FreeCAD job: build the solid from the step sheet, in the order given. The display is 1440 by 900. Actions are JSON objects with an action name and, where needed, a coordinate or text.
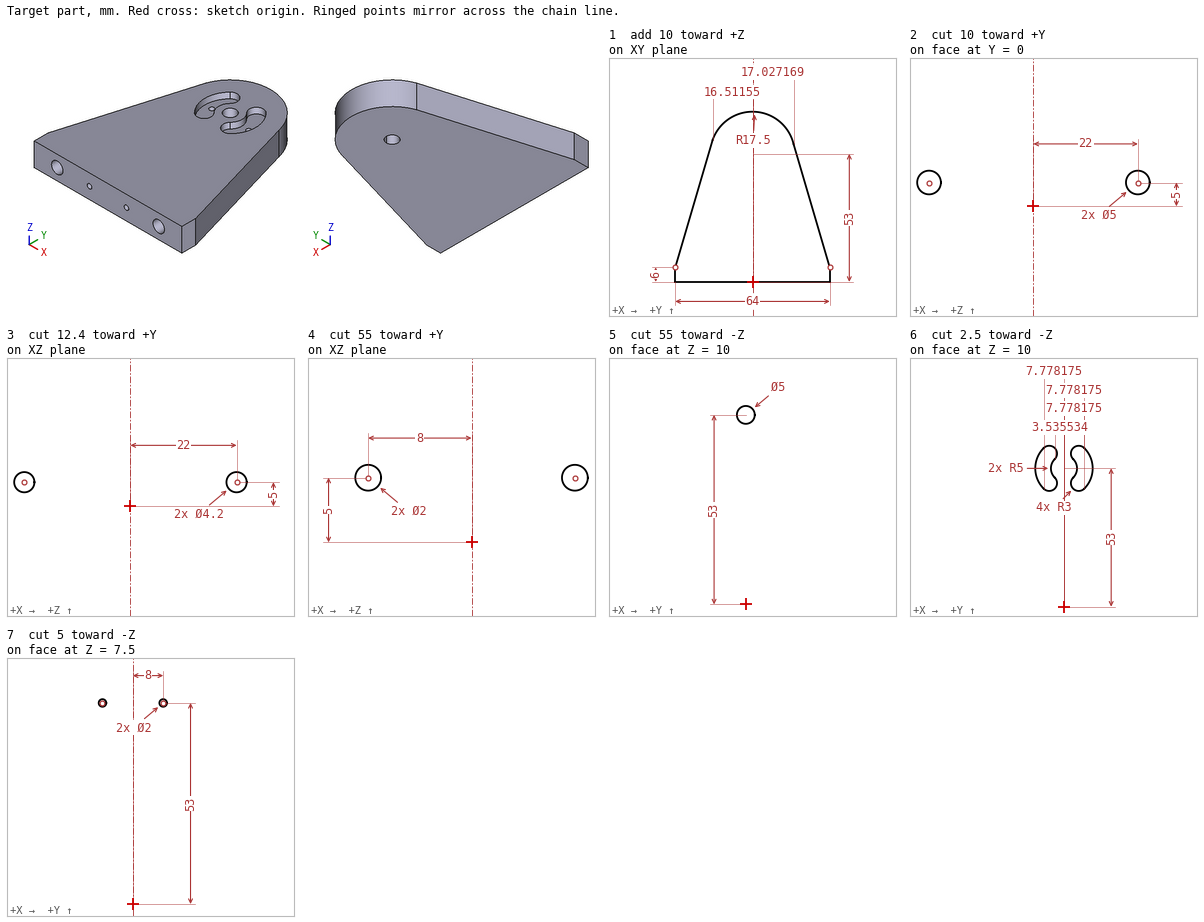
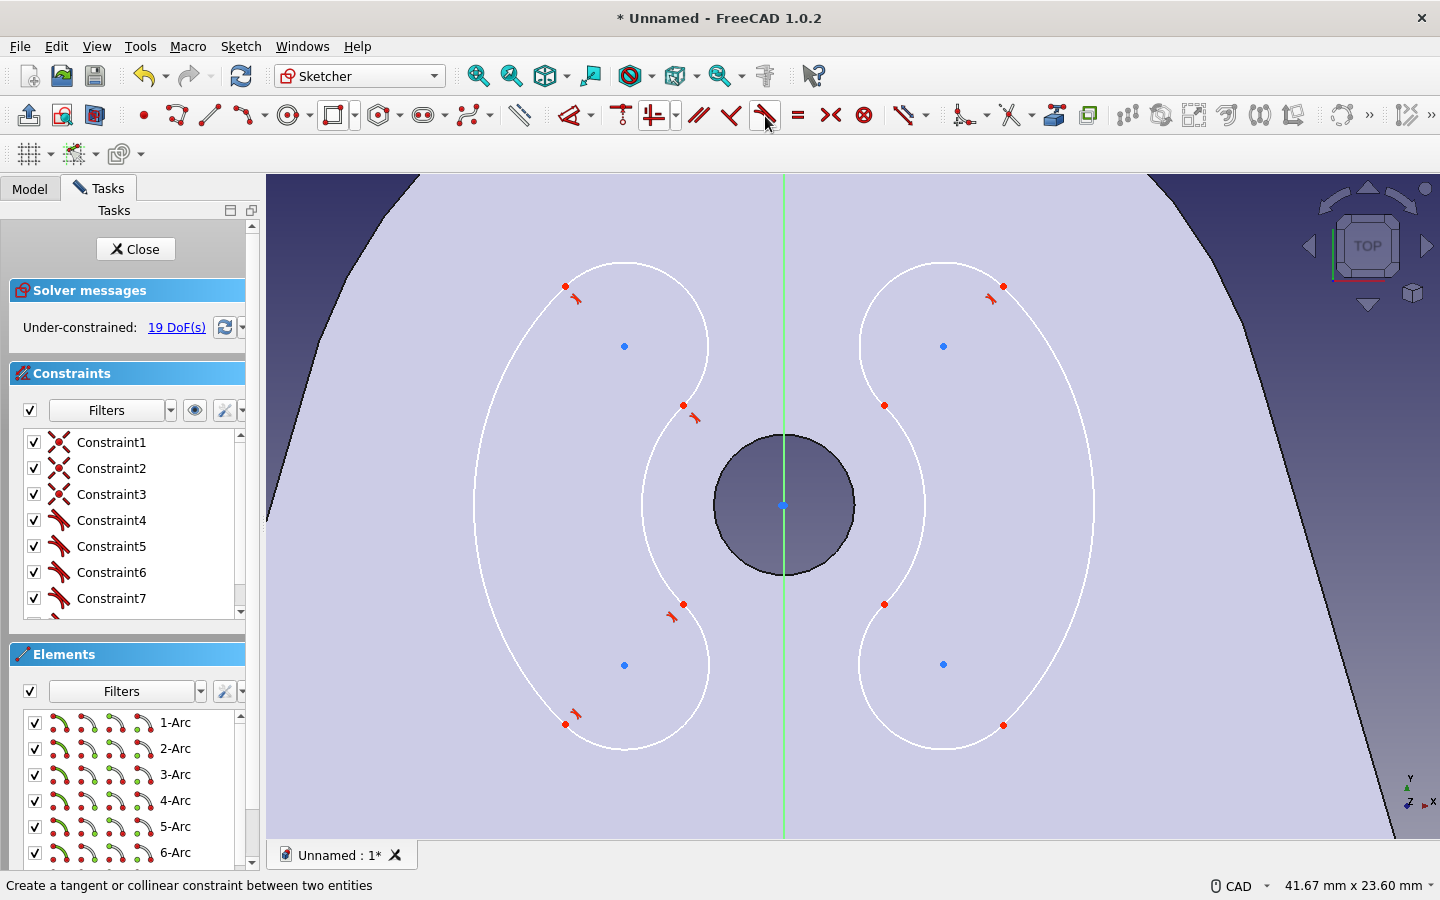
{"action": "left_click", "coordinate": [1079, 602]}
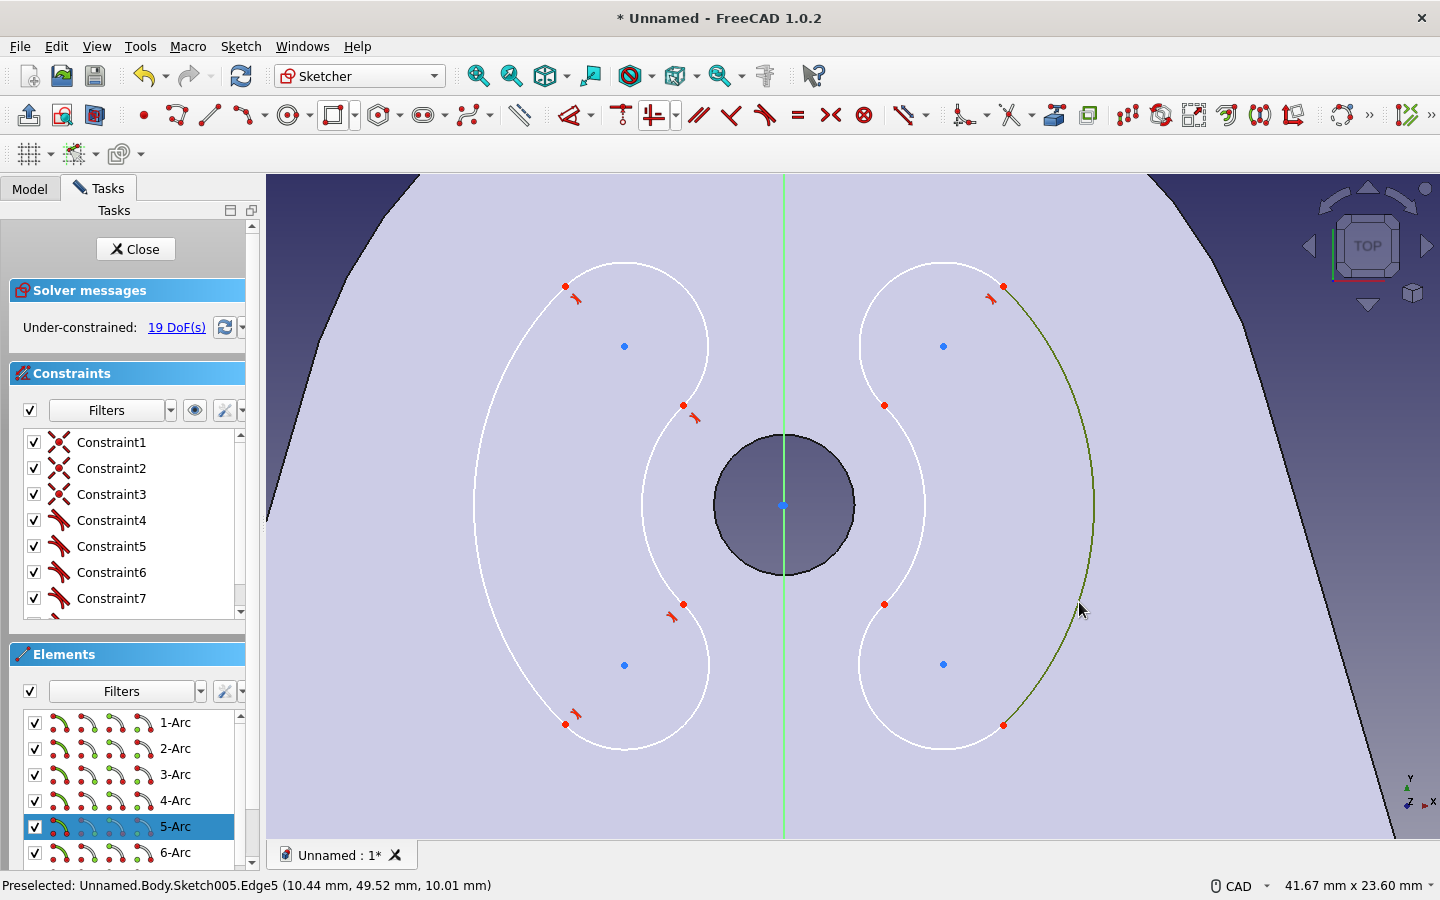
{"action": "left_click", "coordinate": [860, 678]}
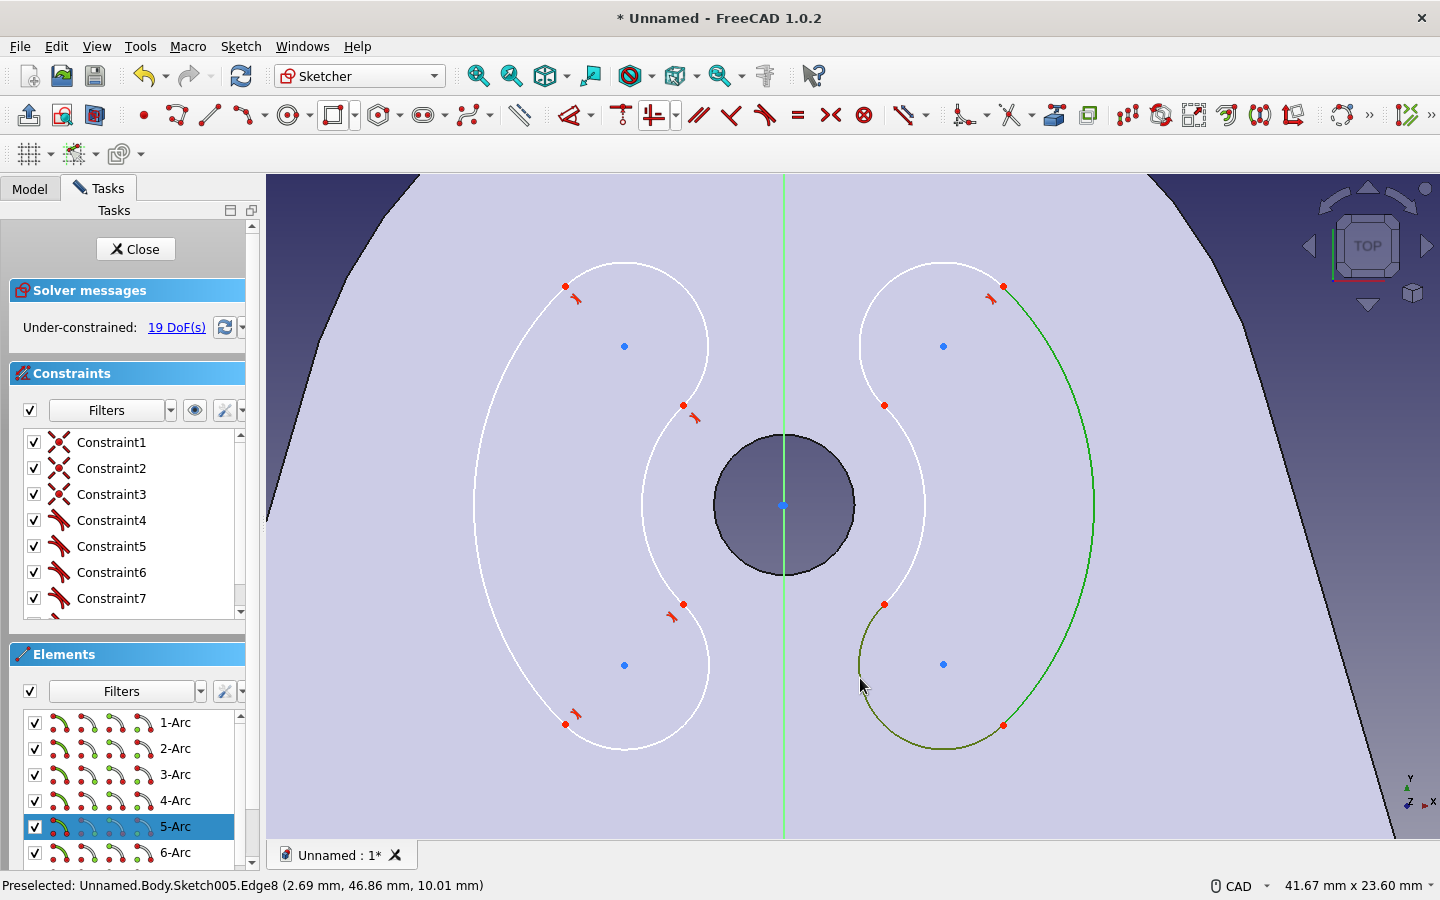
{"action": "left_click", "coordinate": [765, 116]}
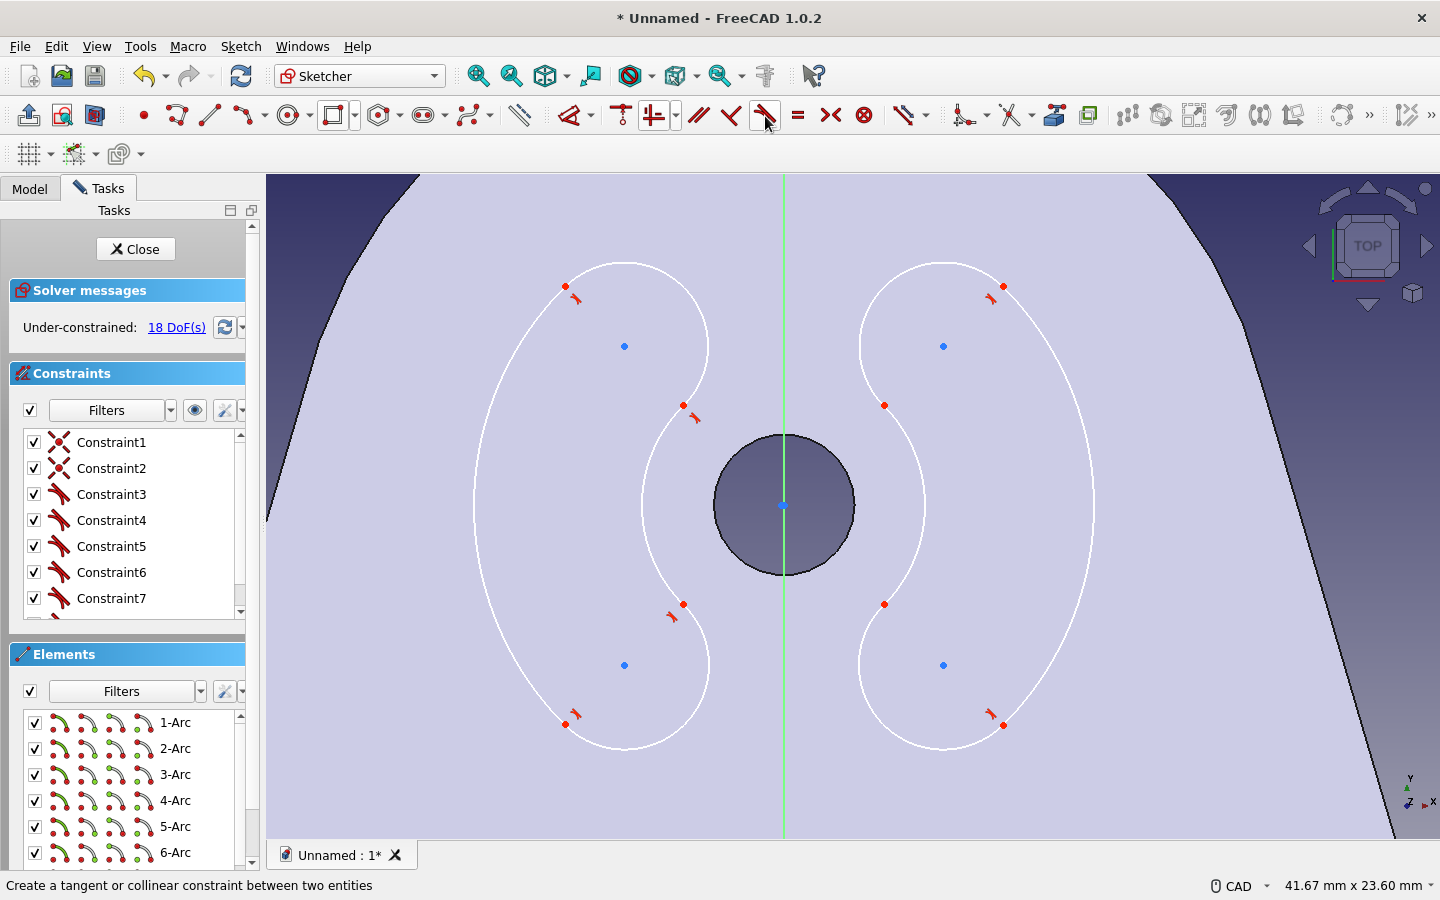
{"action": "left_click", "coordinate": [930, 264]}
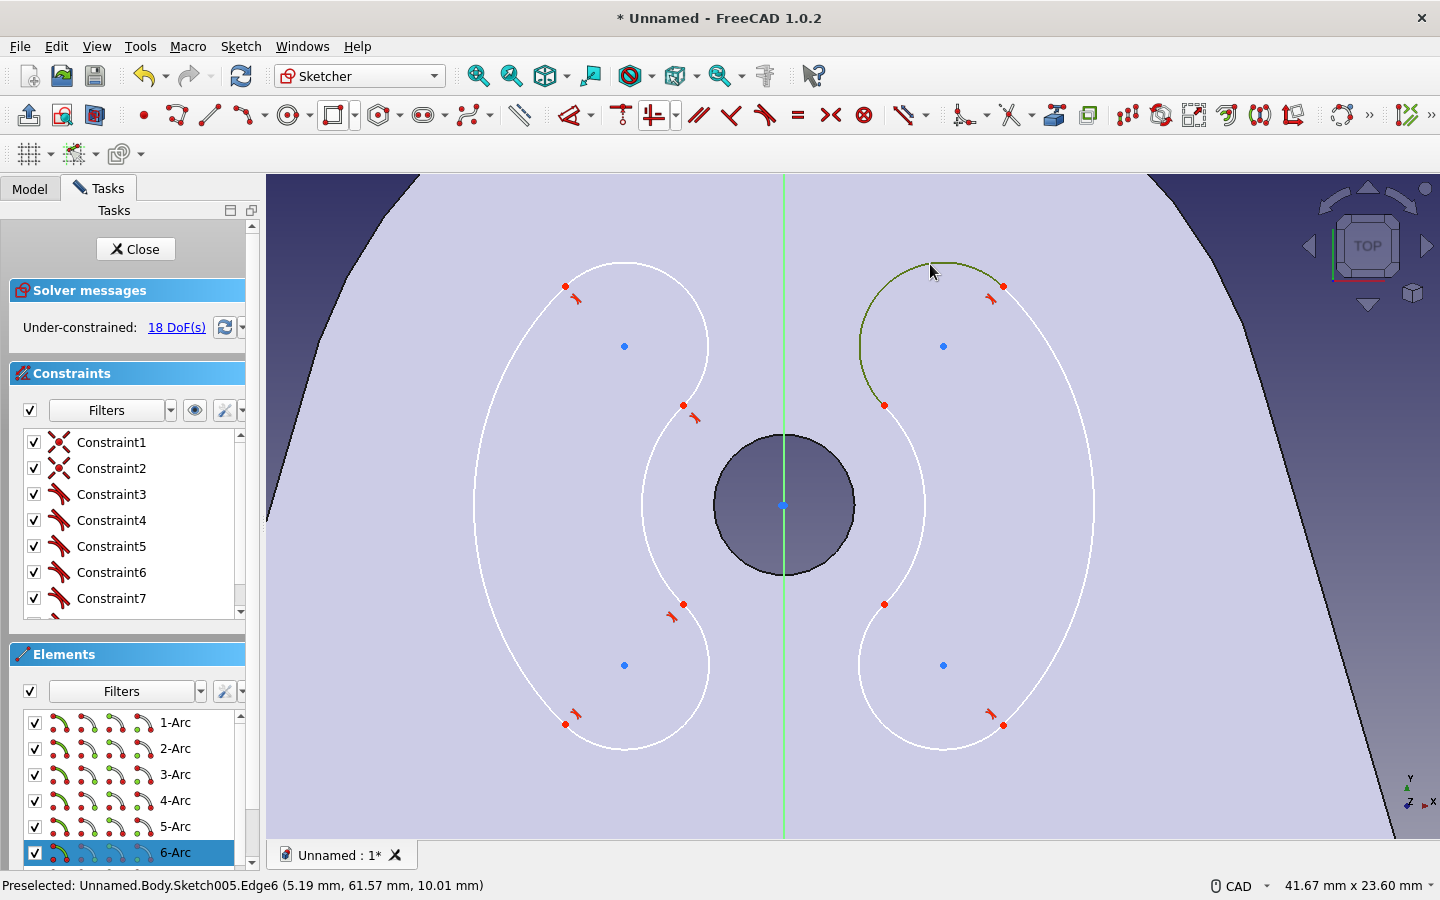
{"action": "left_click", "coordinate": [918, 549]}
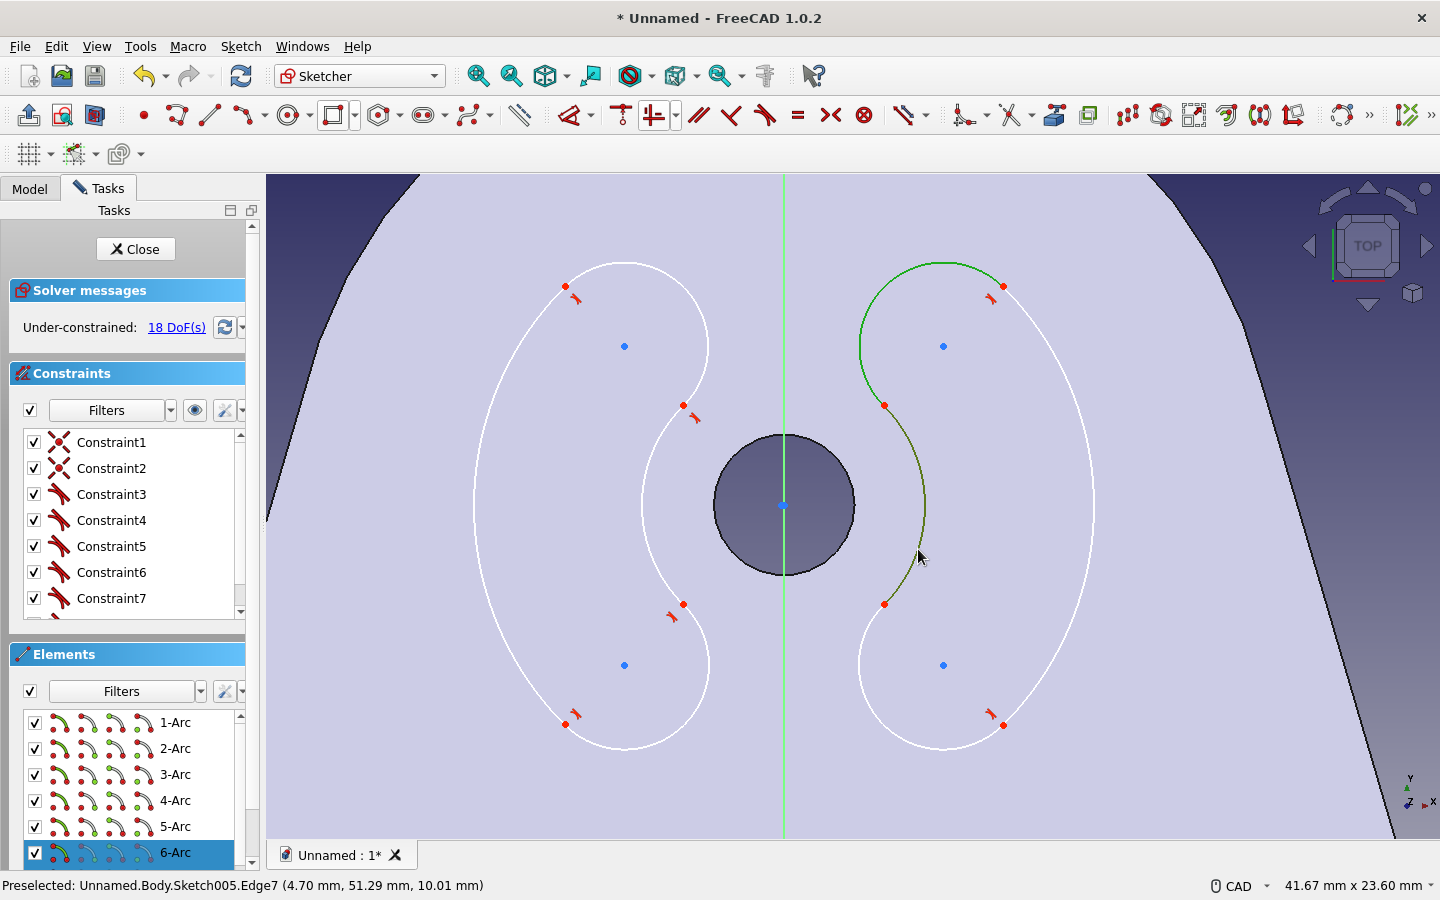
{"action": "left_click", "coordinate": [765, 116]}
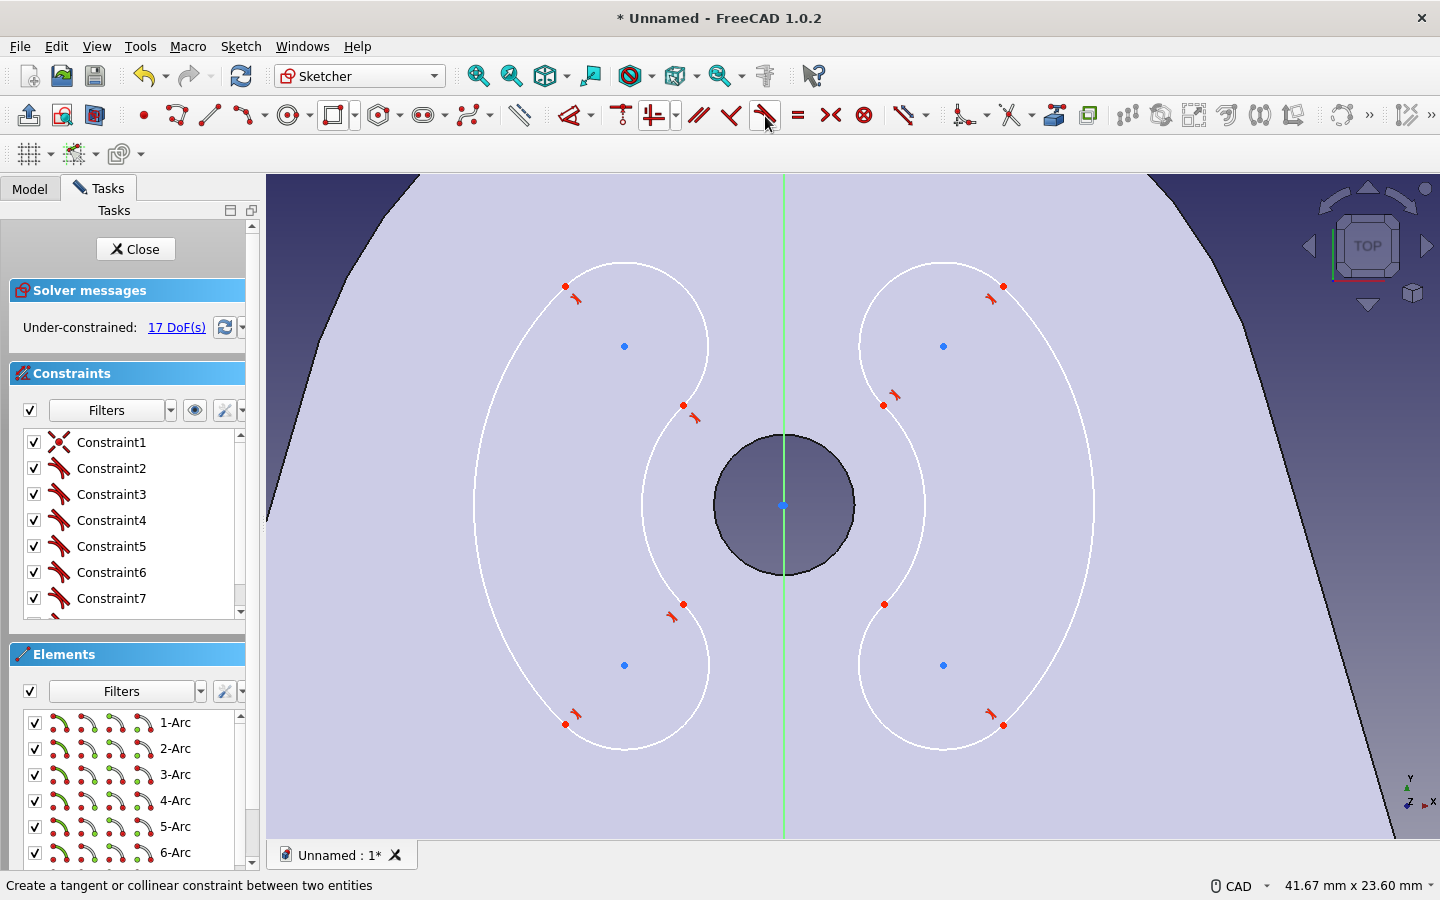
{"action": "left_click", "coordinate": [918, 549]}